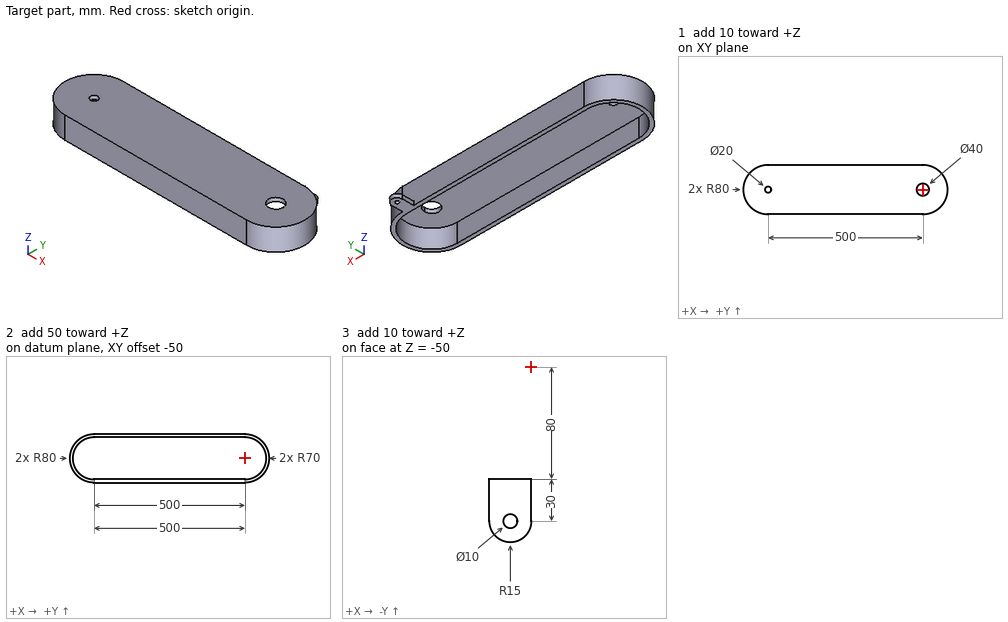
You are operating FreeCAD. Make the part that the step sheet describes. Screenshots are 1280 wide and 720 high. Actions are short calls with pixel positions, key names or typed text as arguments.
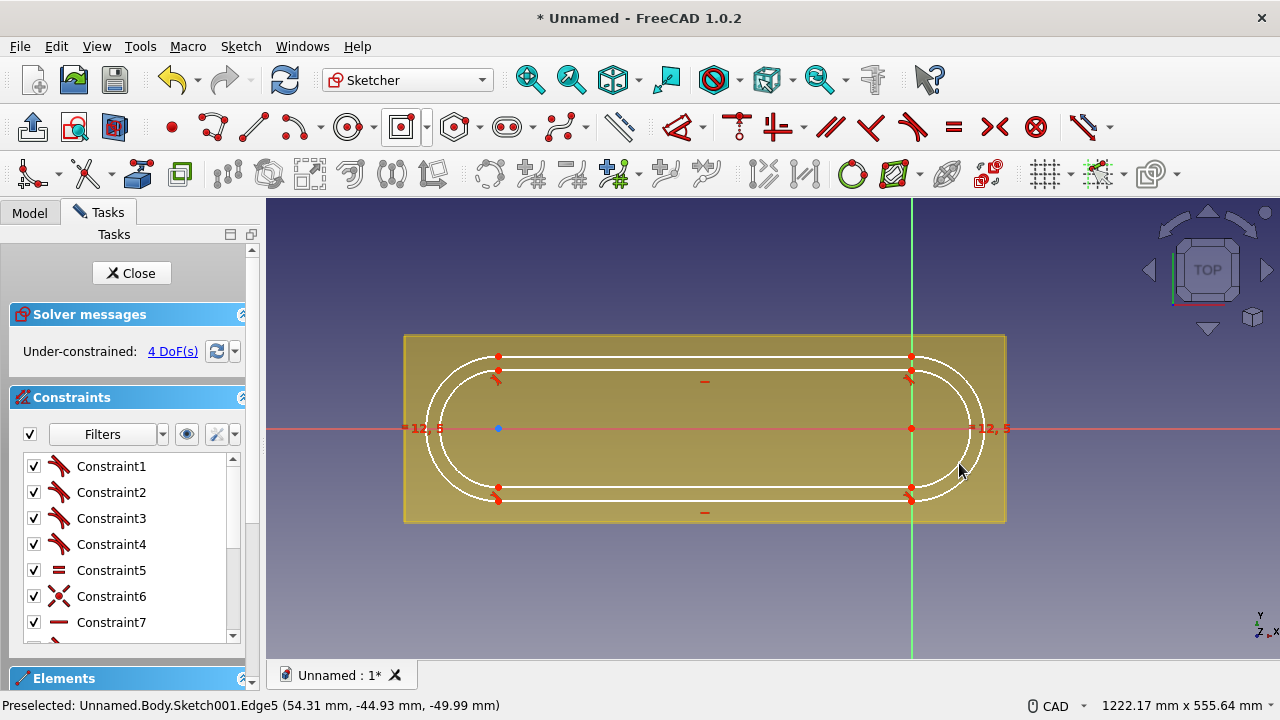
click(676, 128)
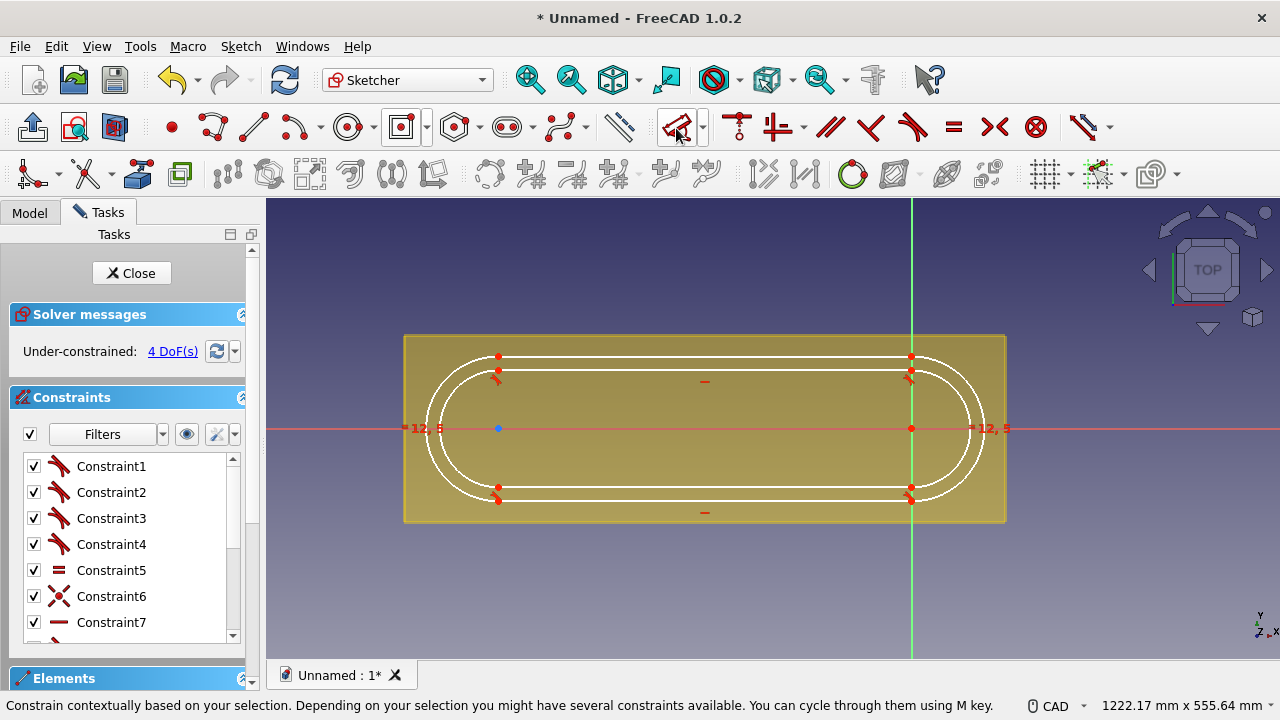
click(971, 471)
click(997, 490)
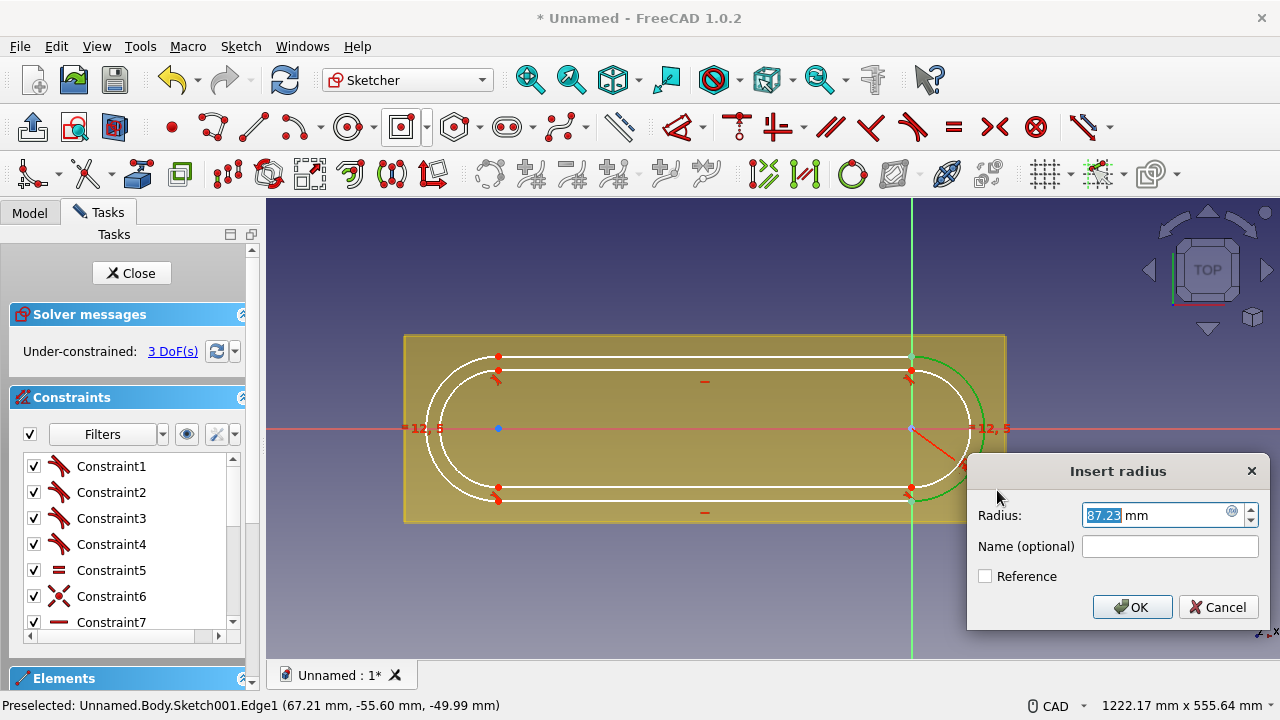
text(80)
key(Return)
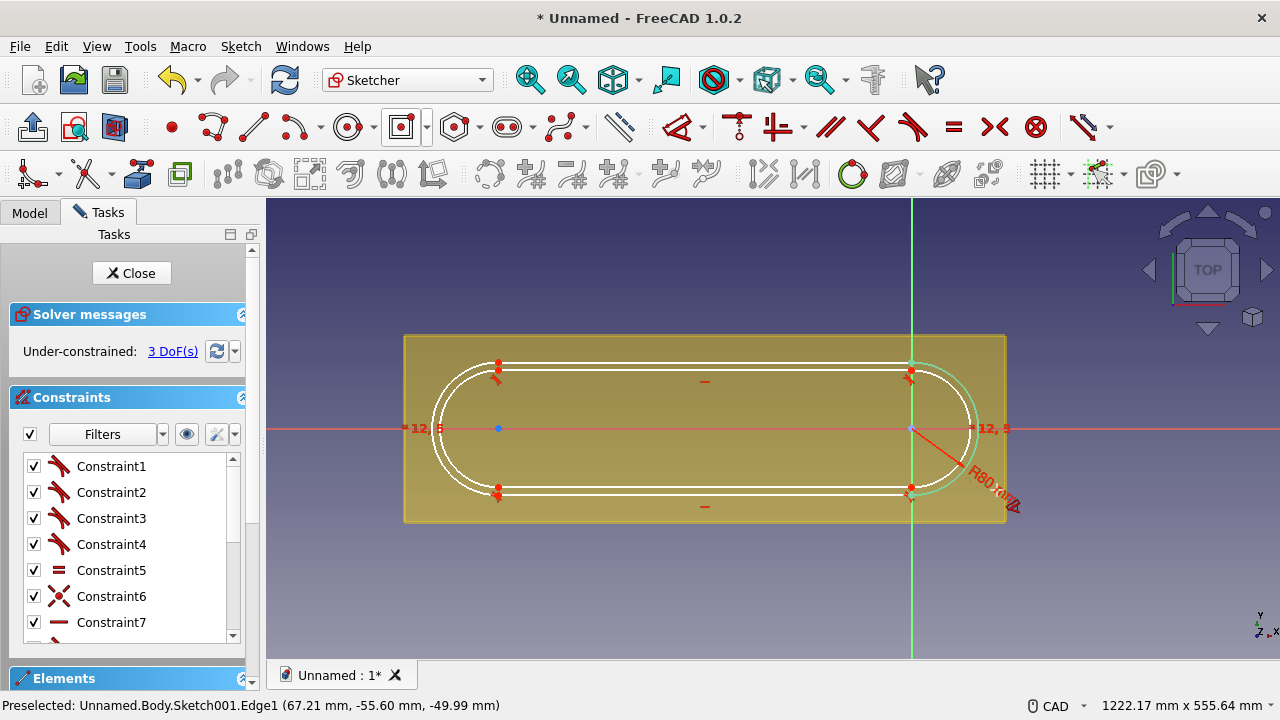
scroll(959, 463, up, 3)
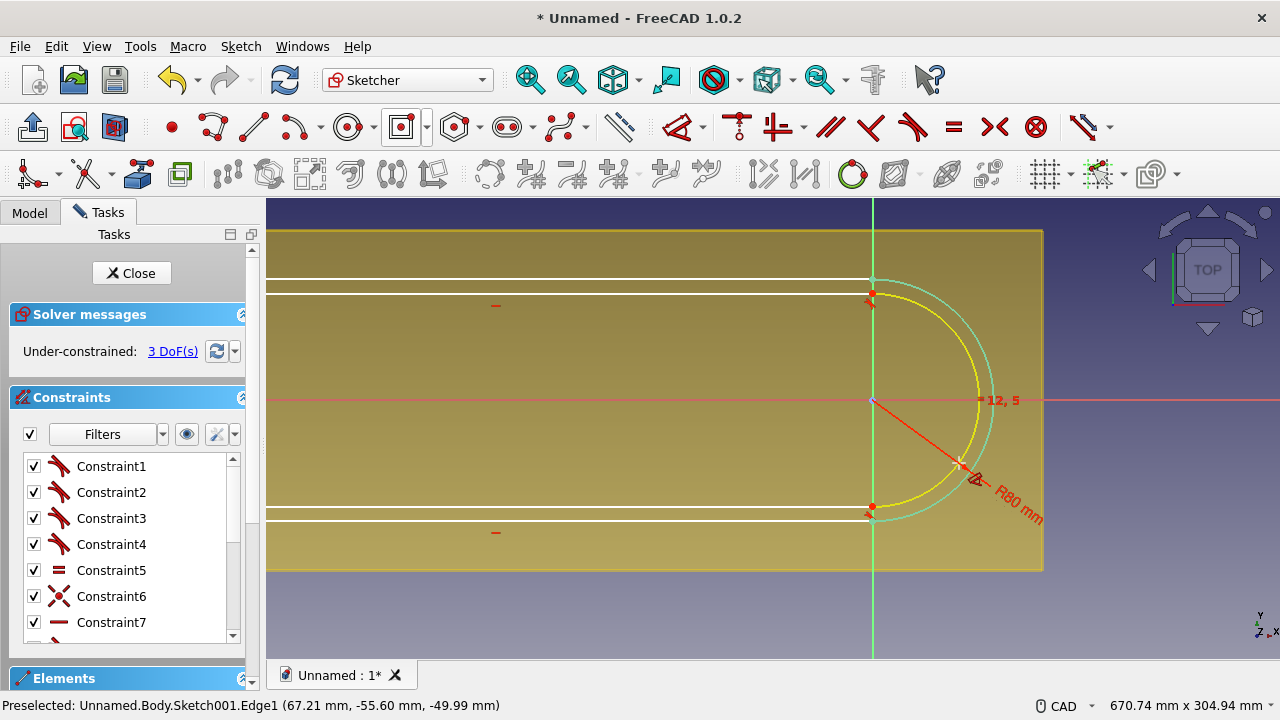
click(959, 463)
click(985, 482)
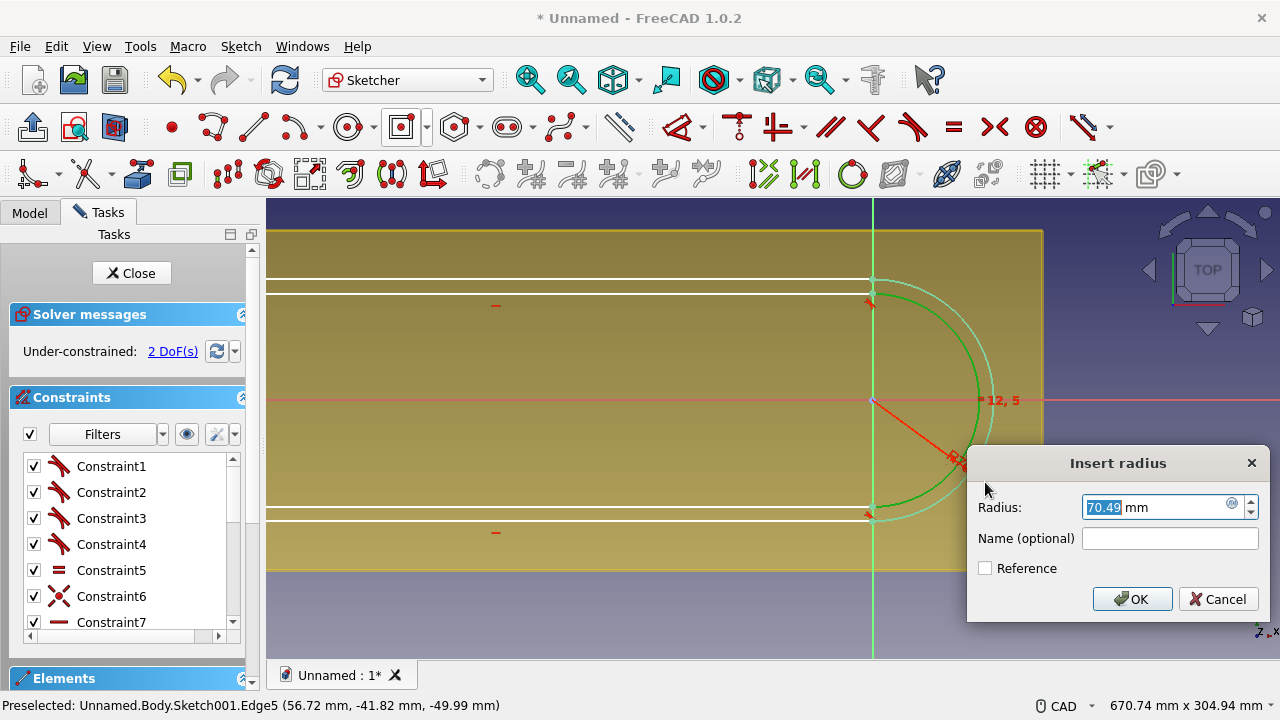
text(70)
key(Return)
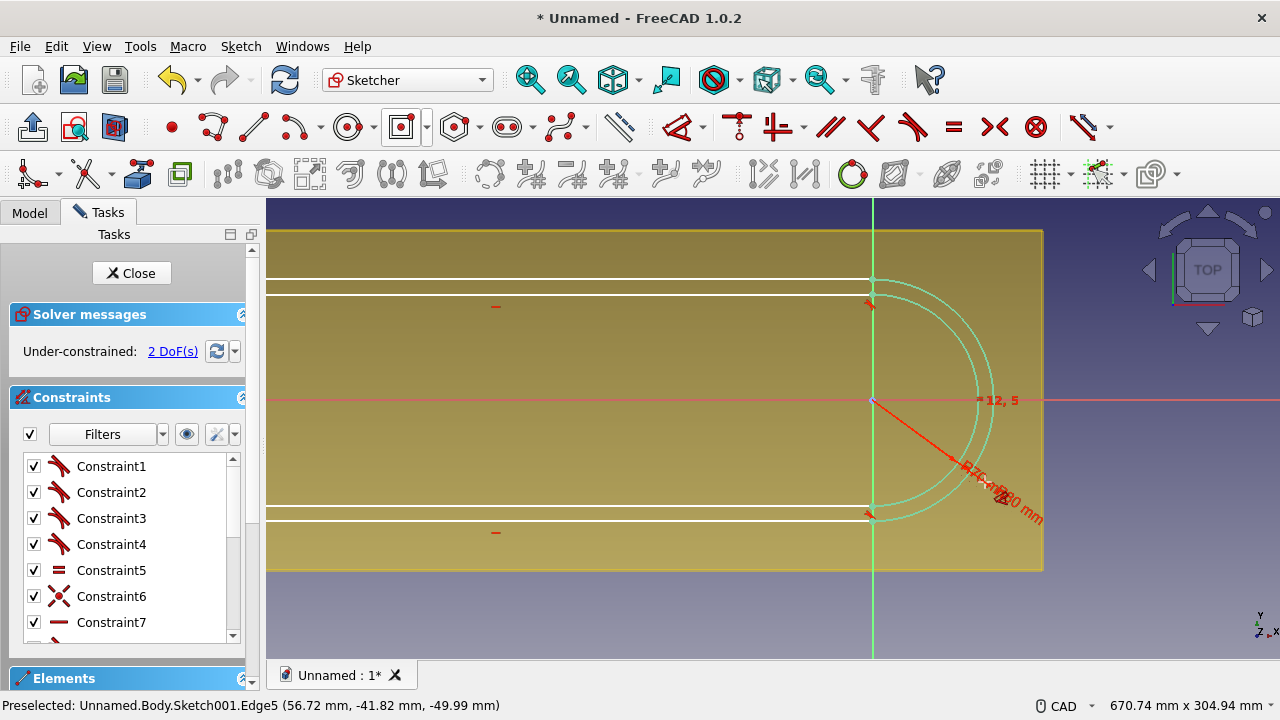
click(647, 521)
click(583, 555)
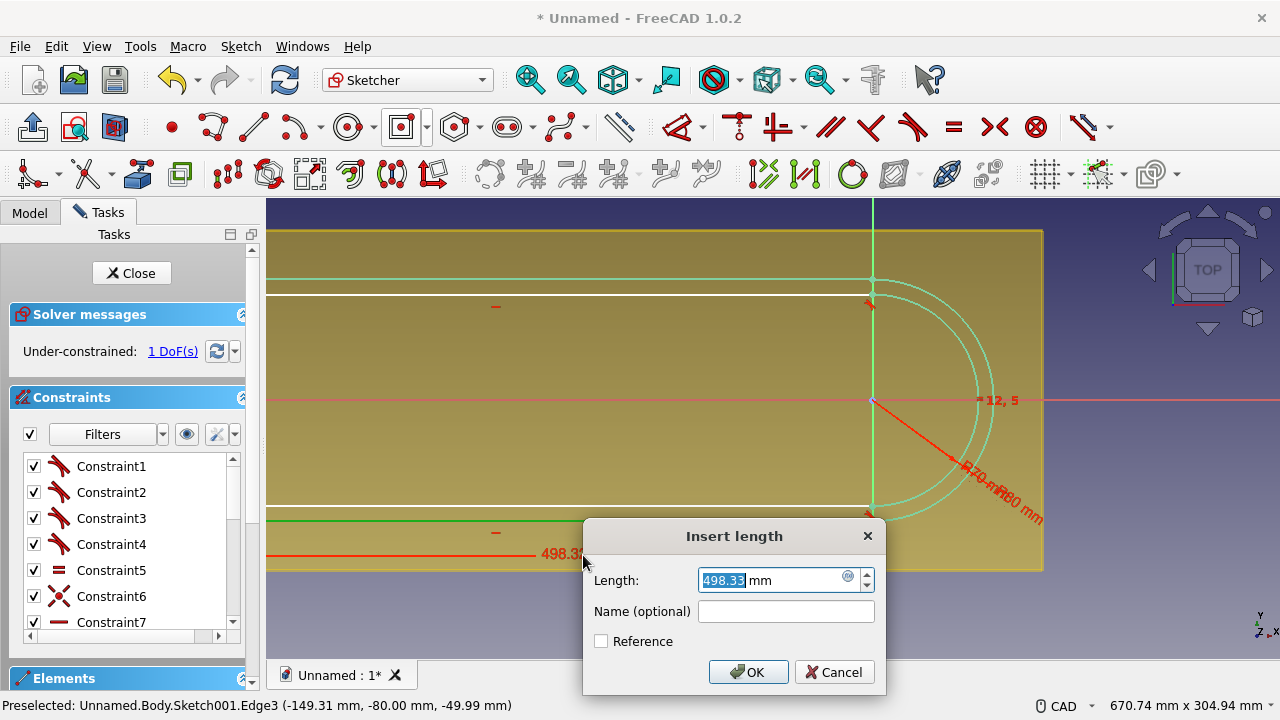
text(500)
key(Return)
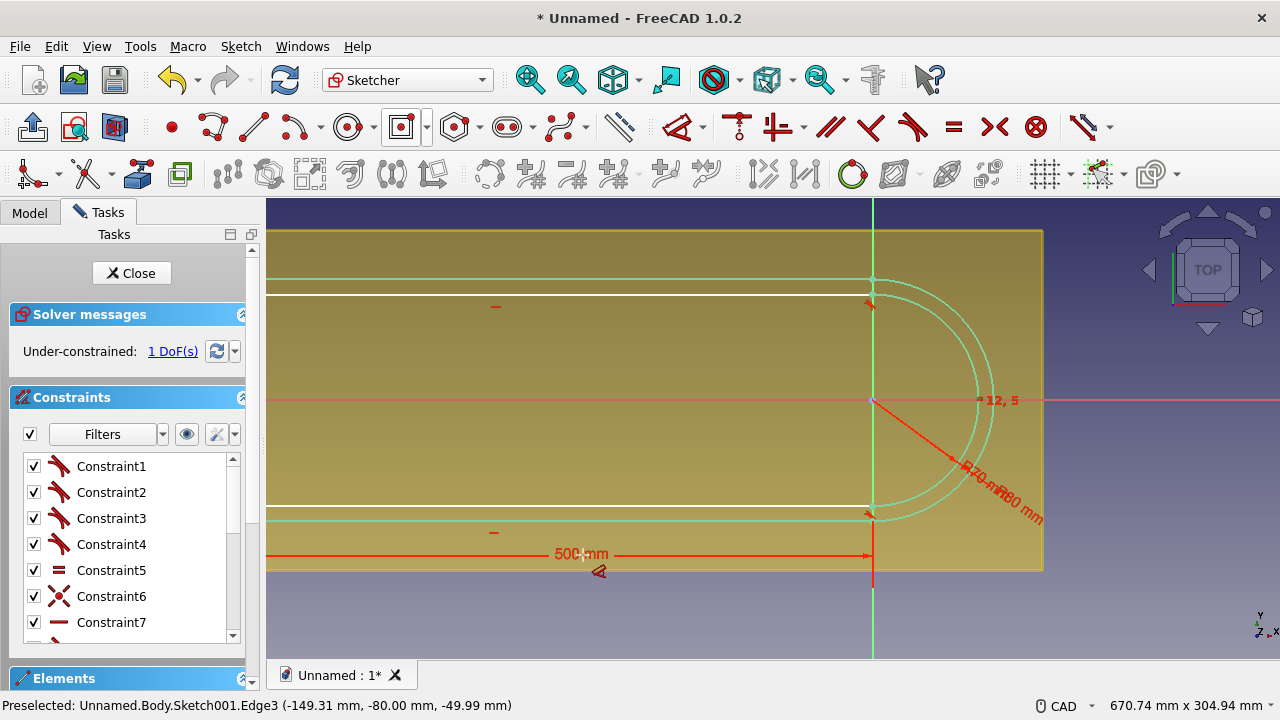
click(647, 506)
click(450, 540)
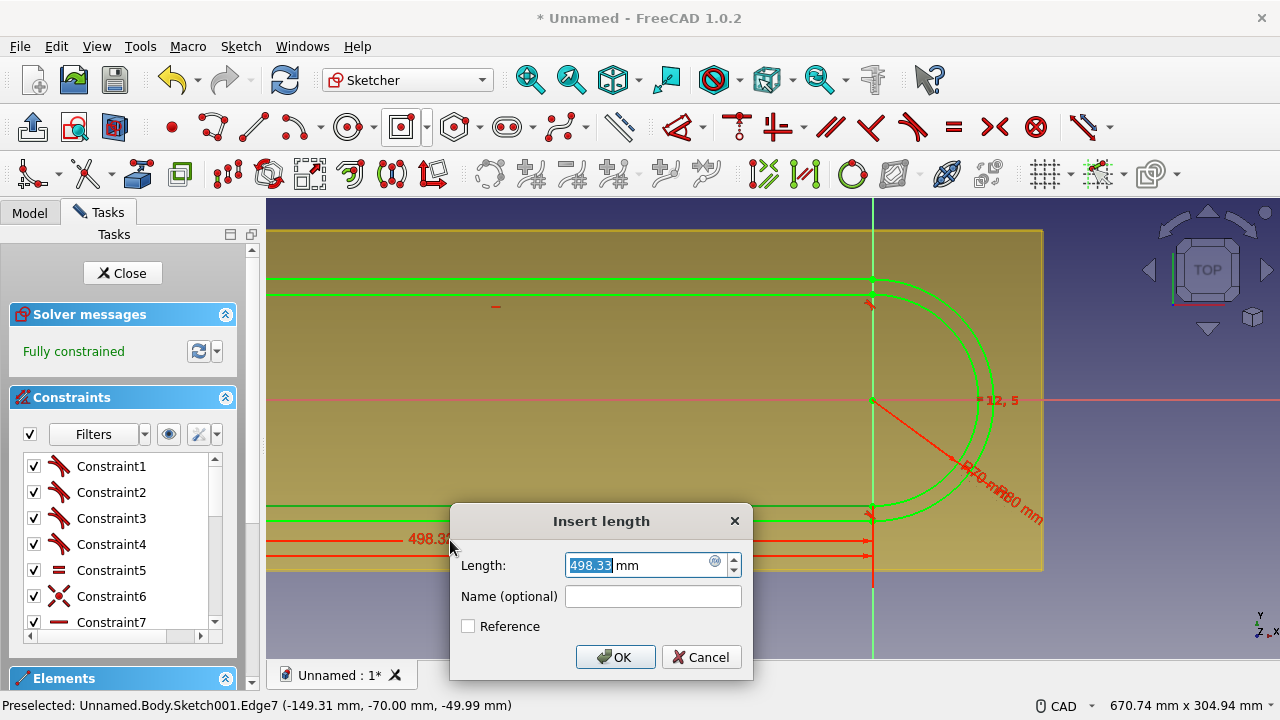
text(500)
key(Return)
key(Escape)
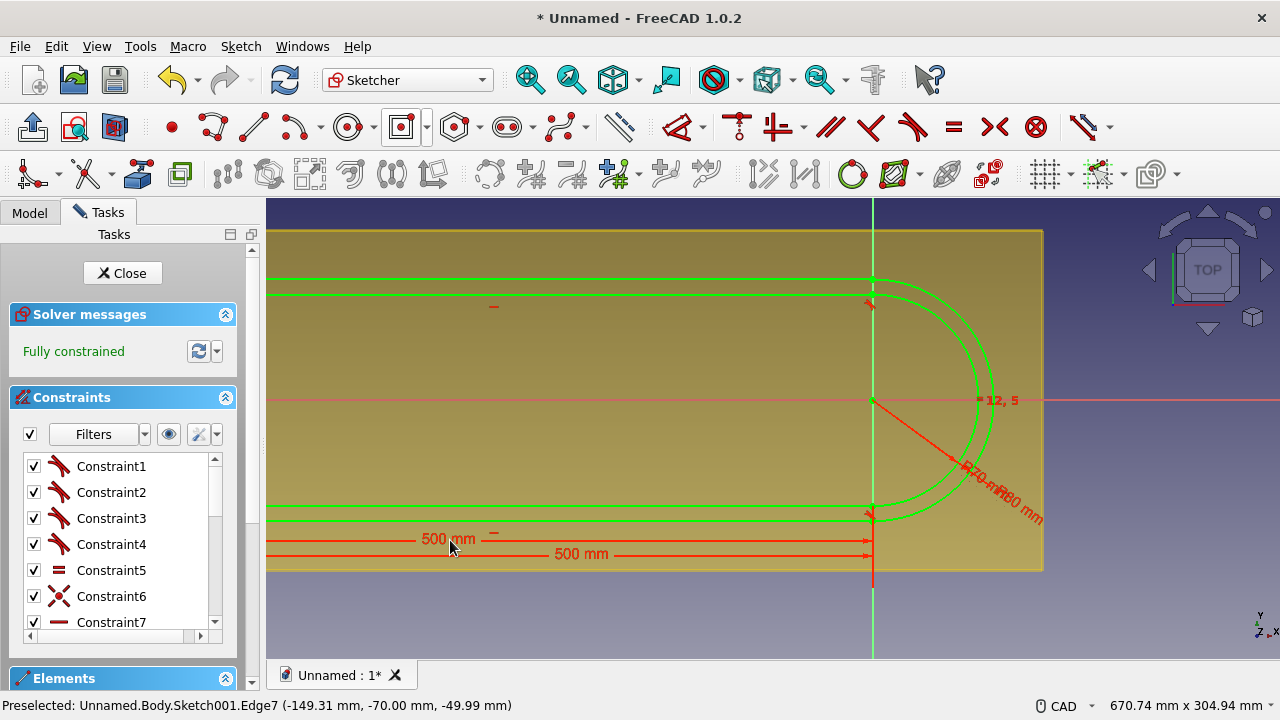
click(123, 273)